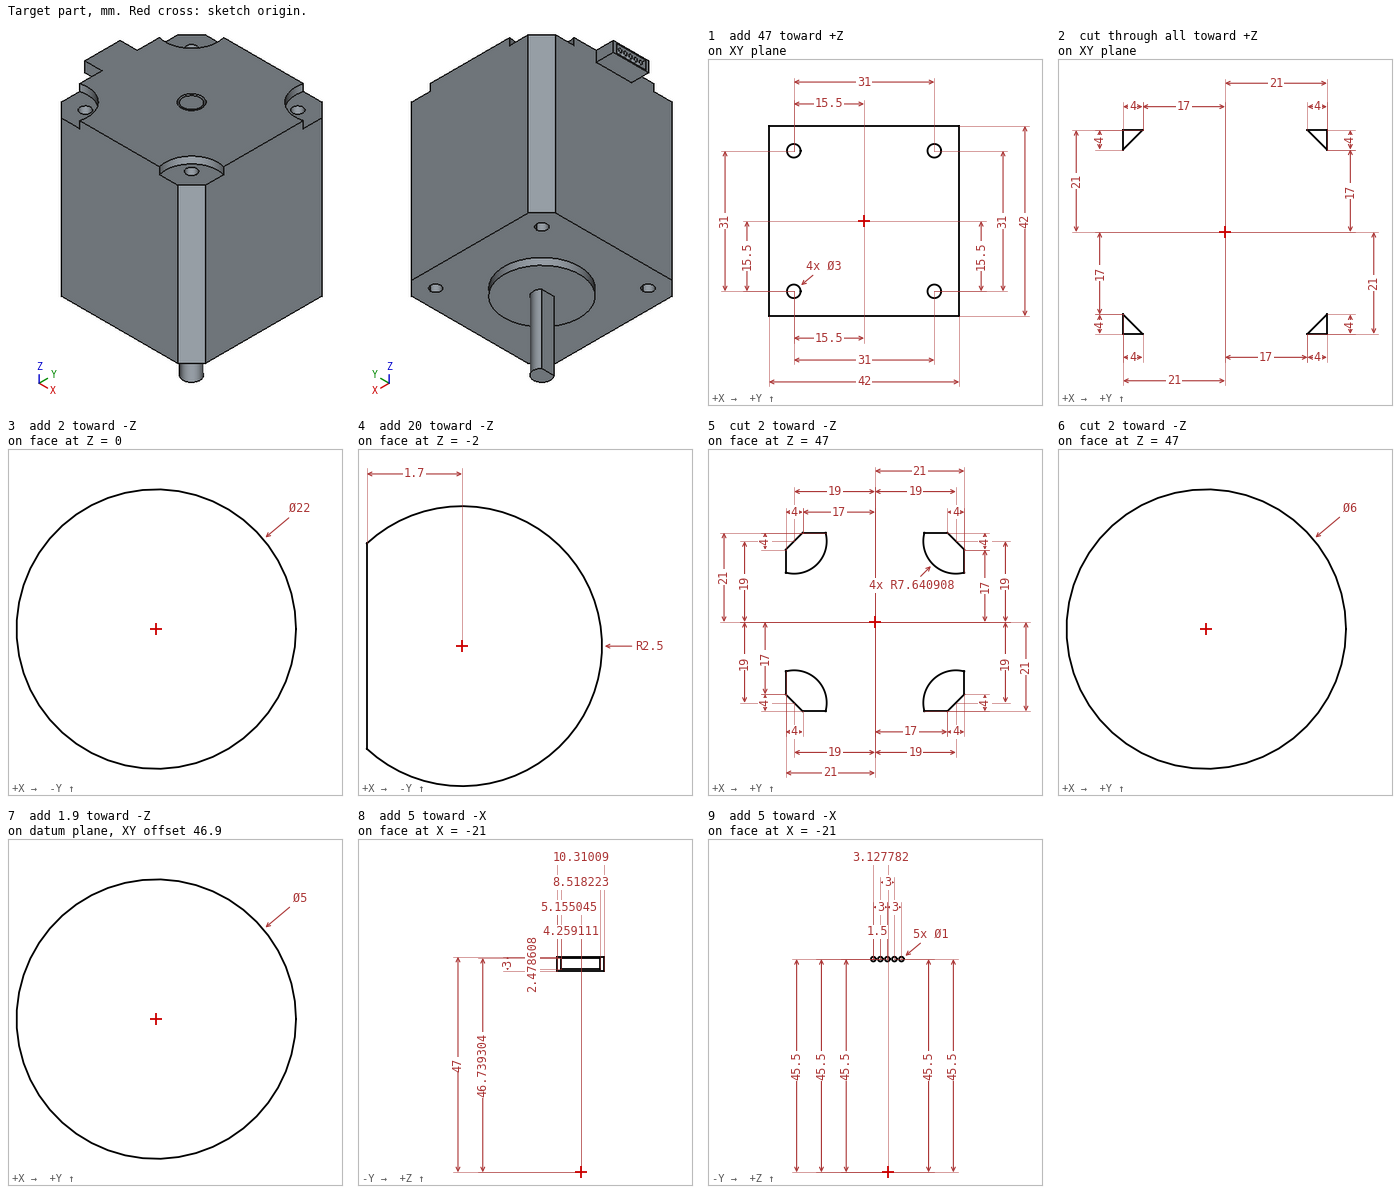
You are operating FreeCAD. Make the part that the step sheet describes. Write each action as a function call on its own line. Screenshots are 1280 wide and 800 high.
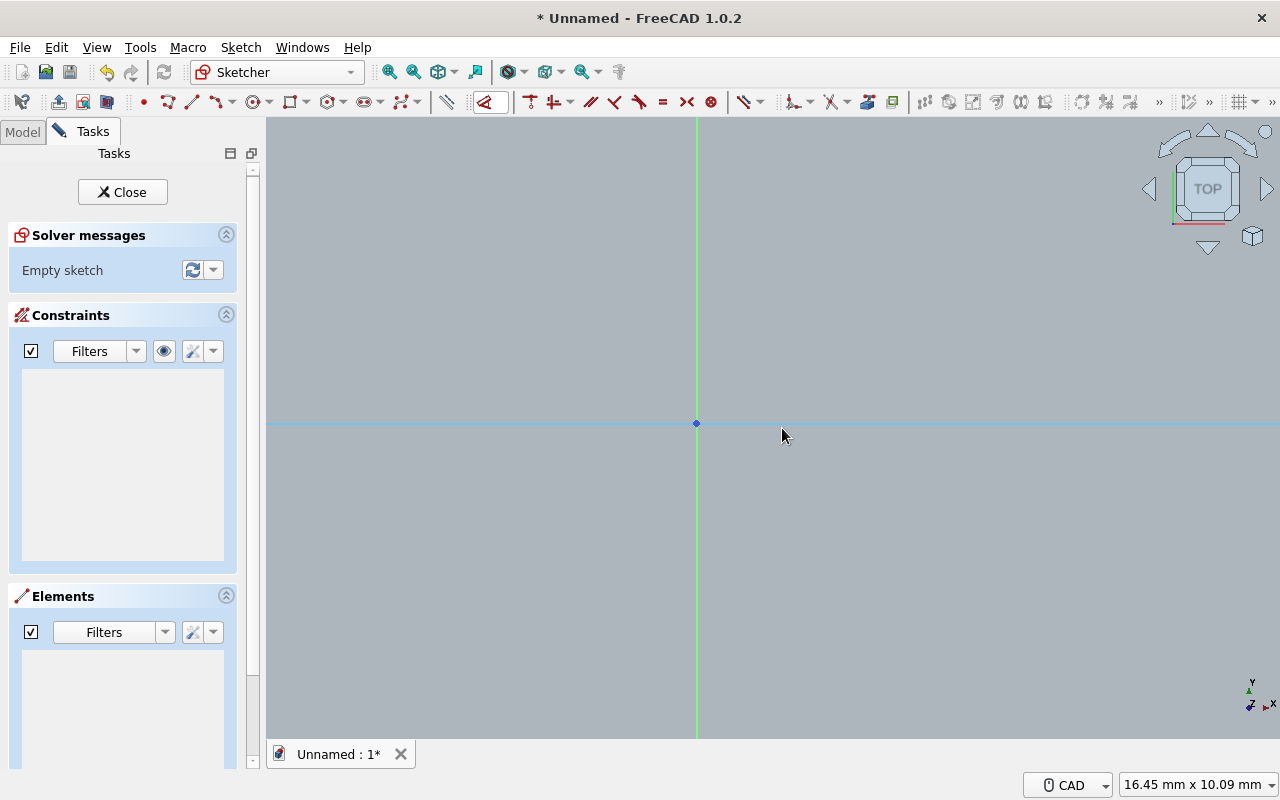
click(254, 102)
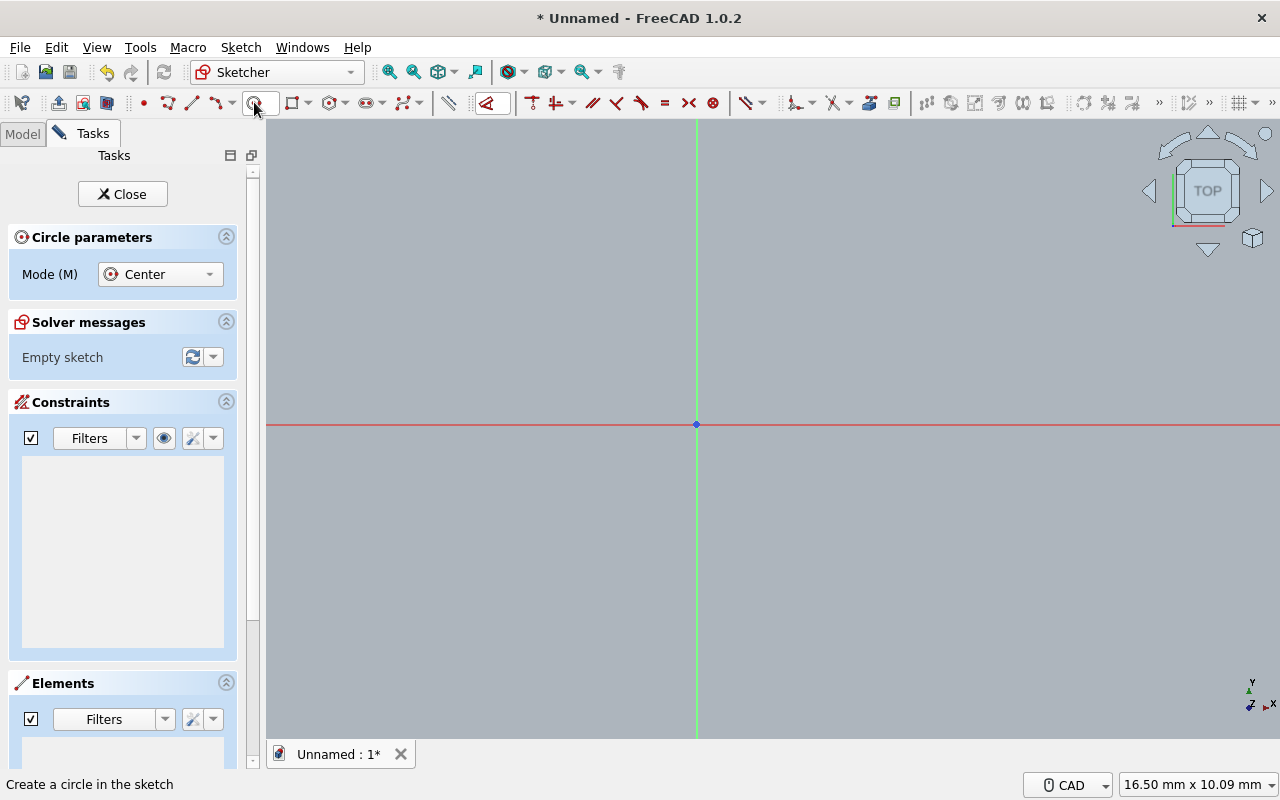
click(697, 425)
click(827, 295)
key(Escape)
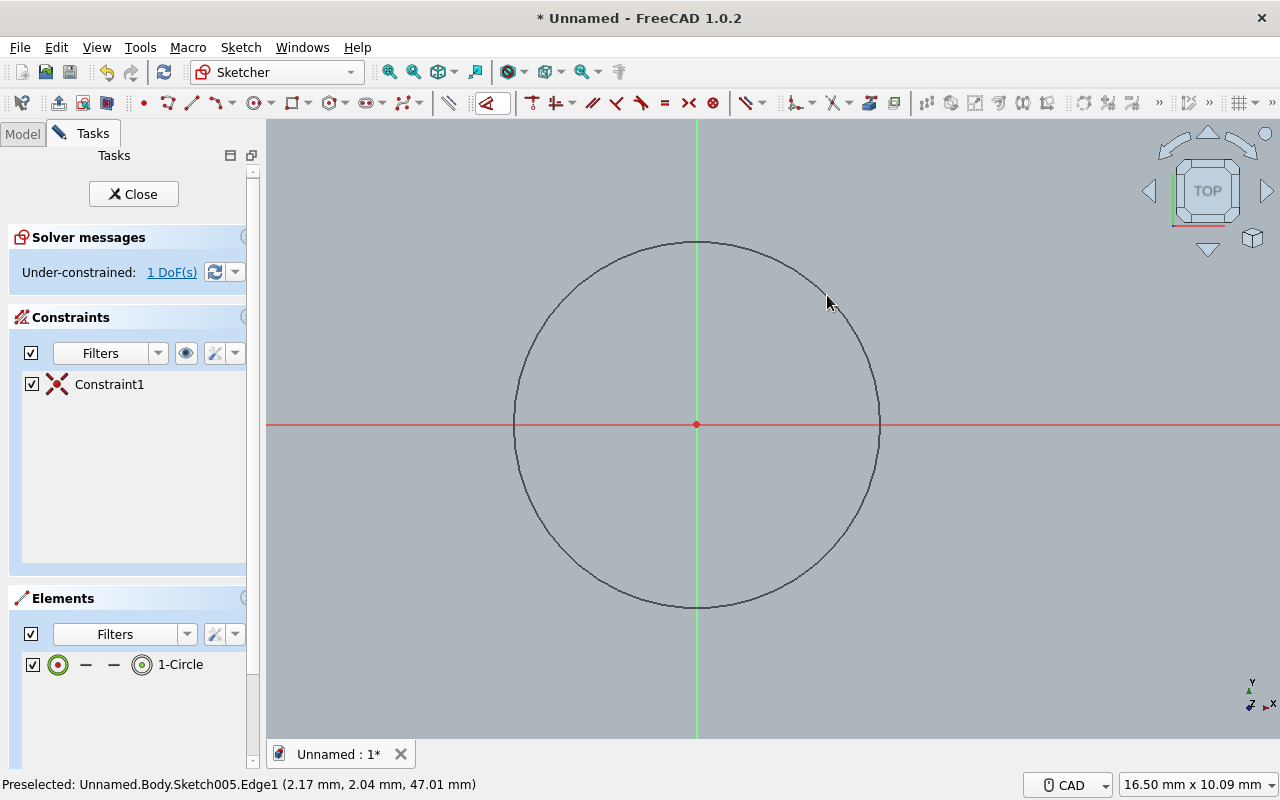
click(826, 295)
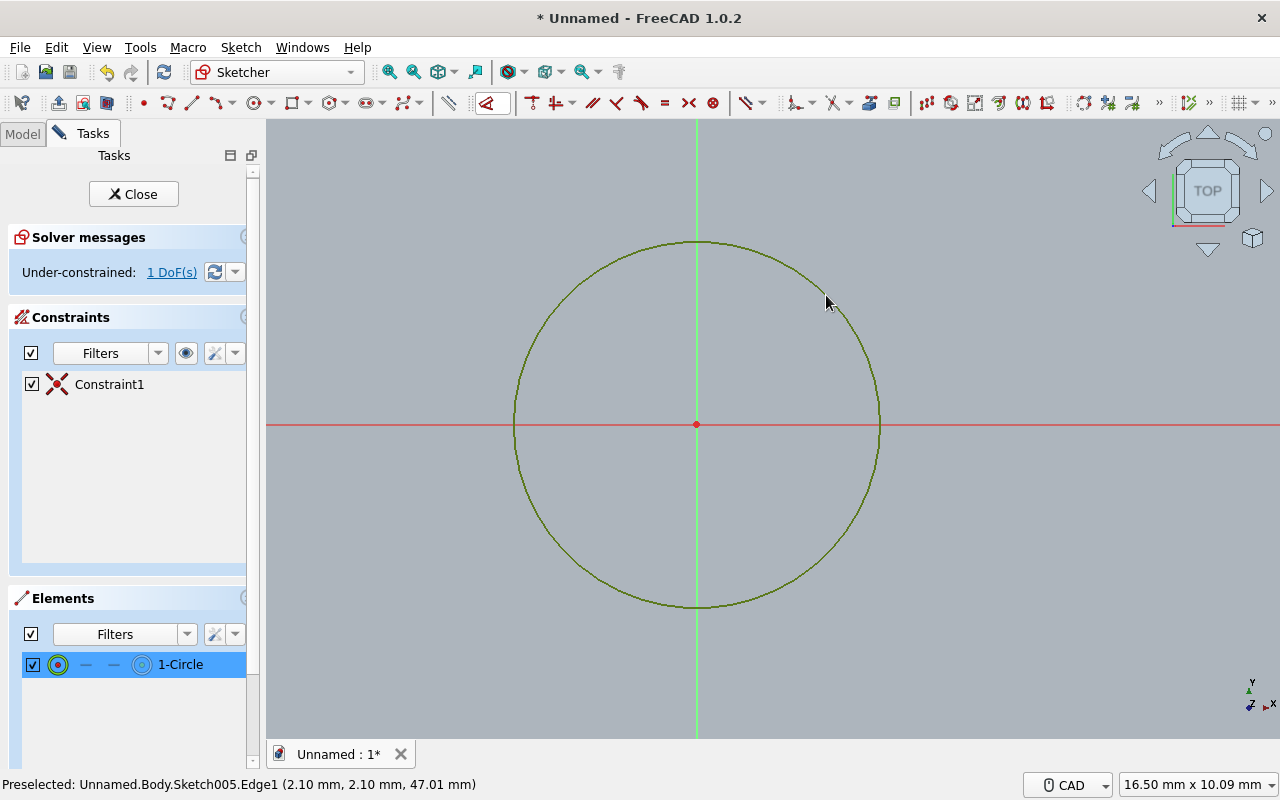
click(504, 104)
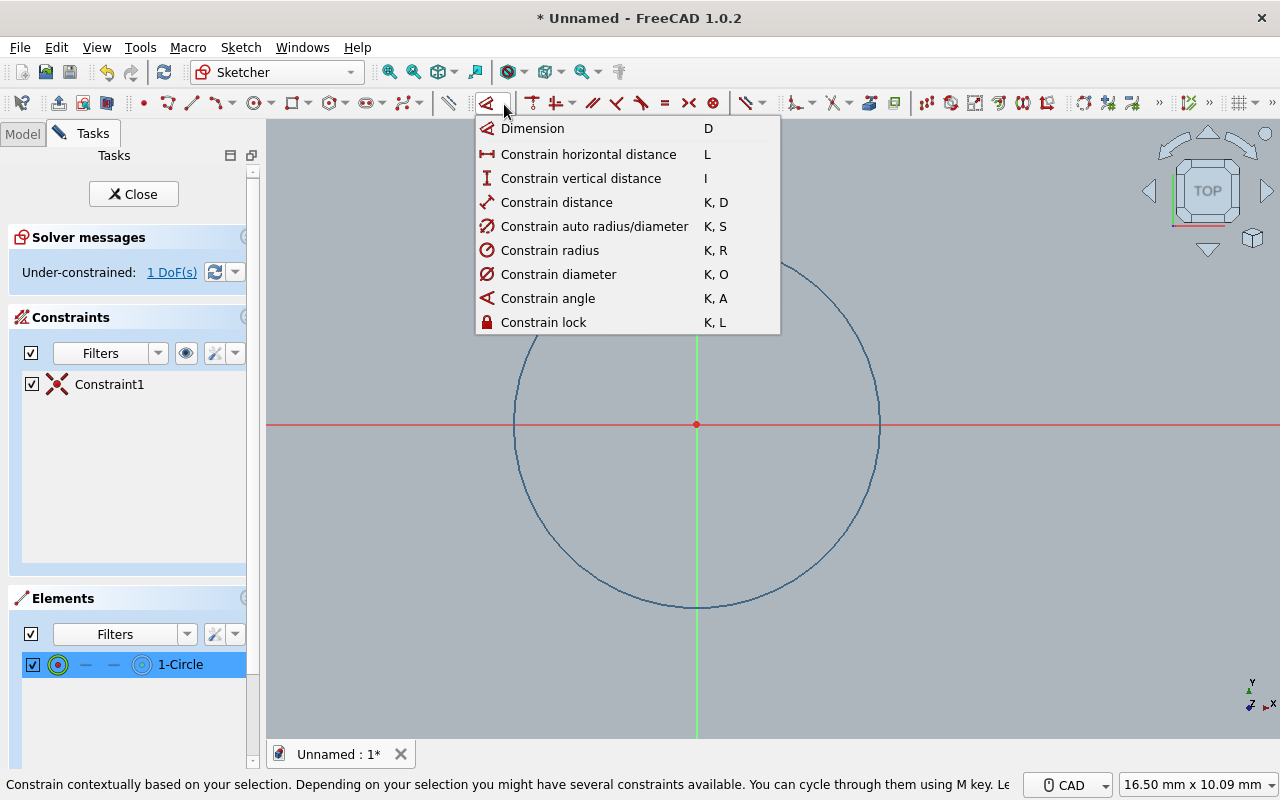
click(628, 274)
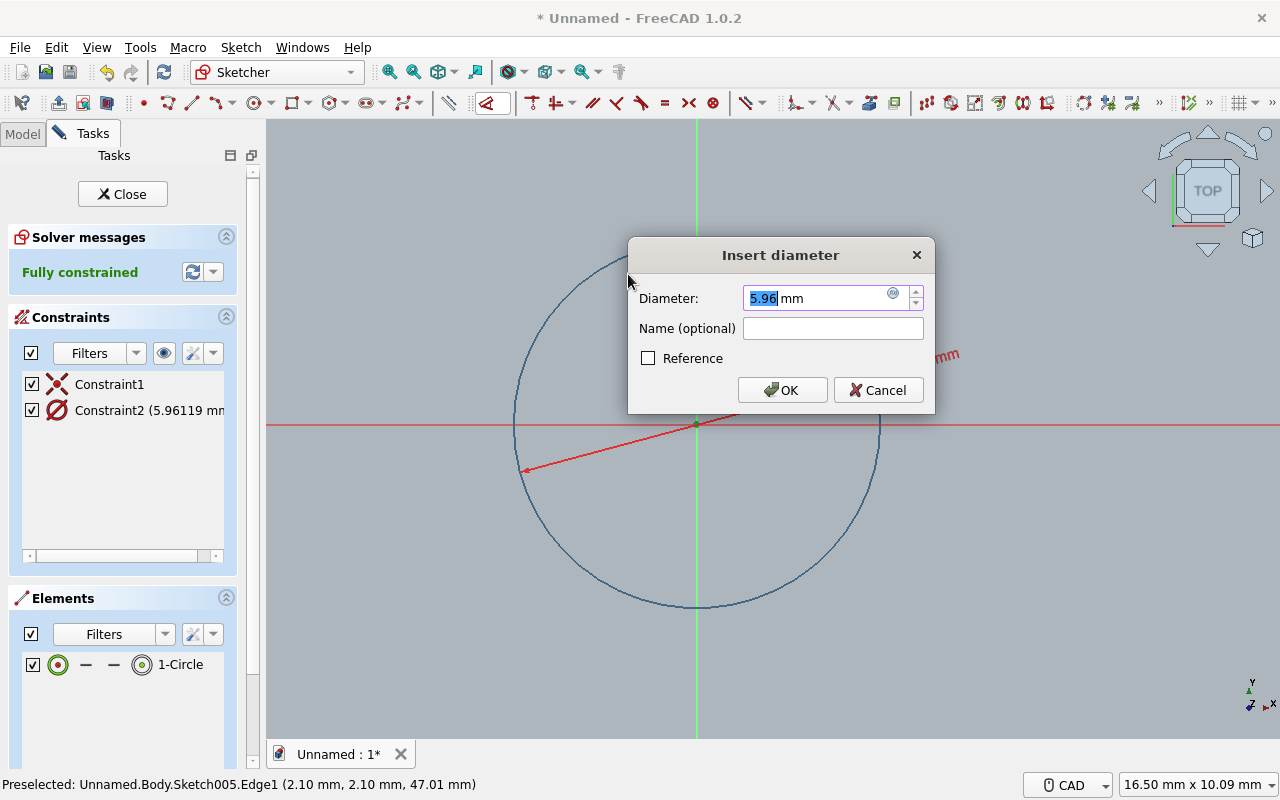
text(6)
key(Return)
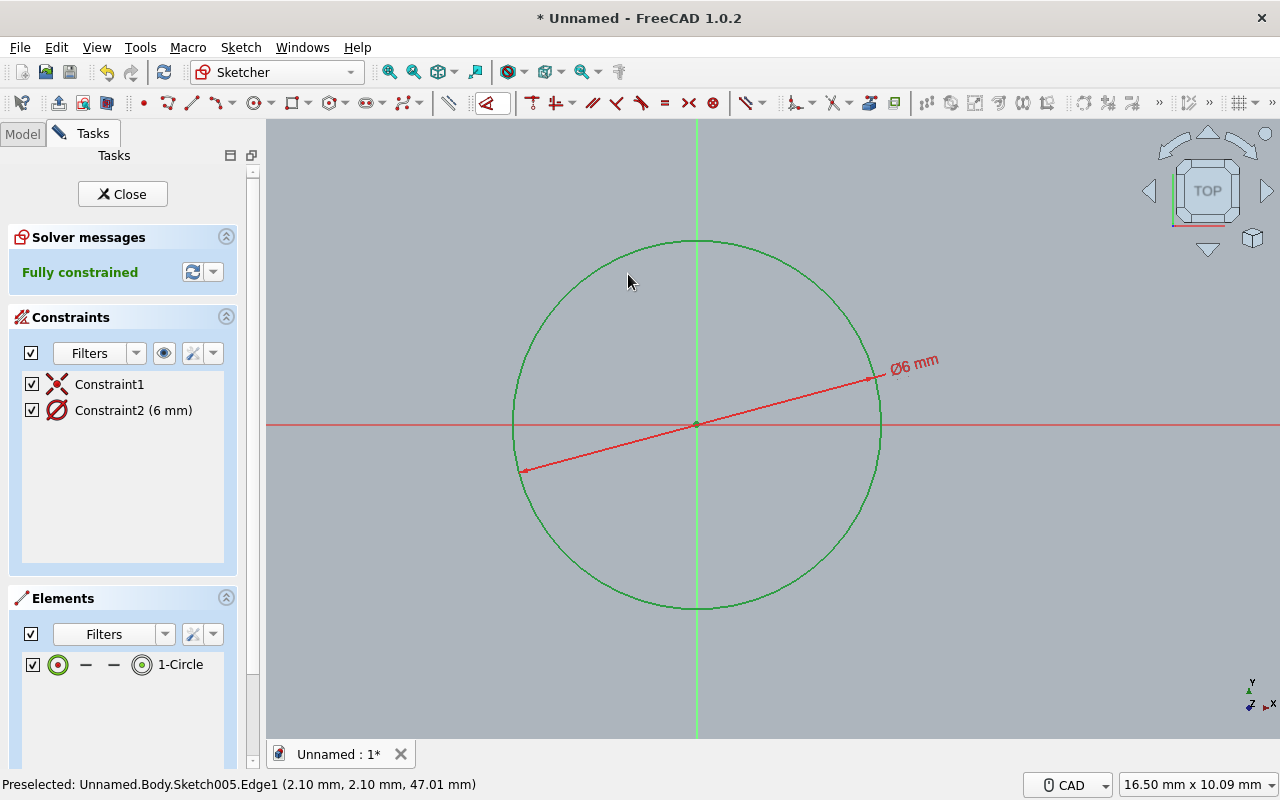
click(123, 194)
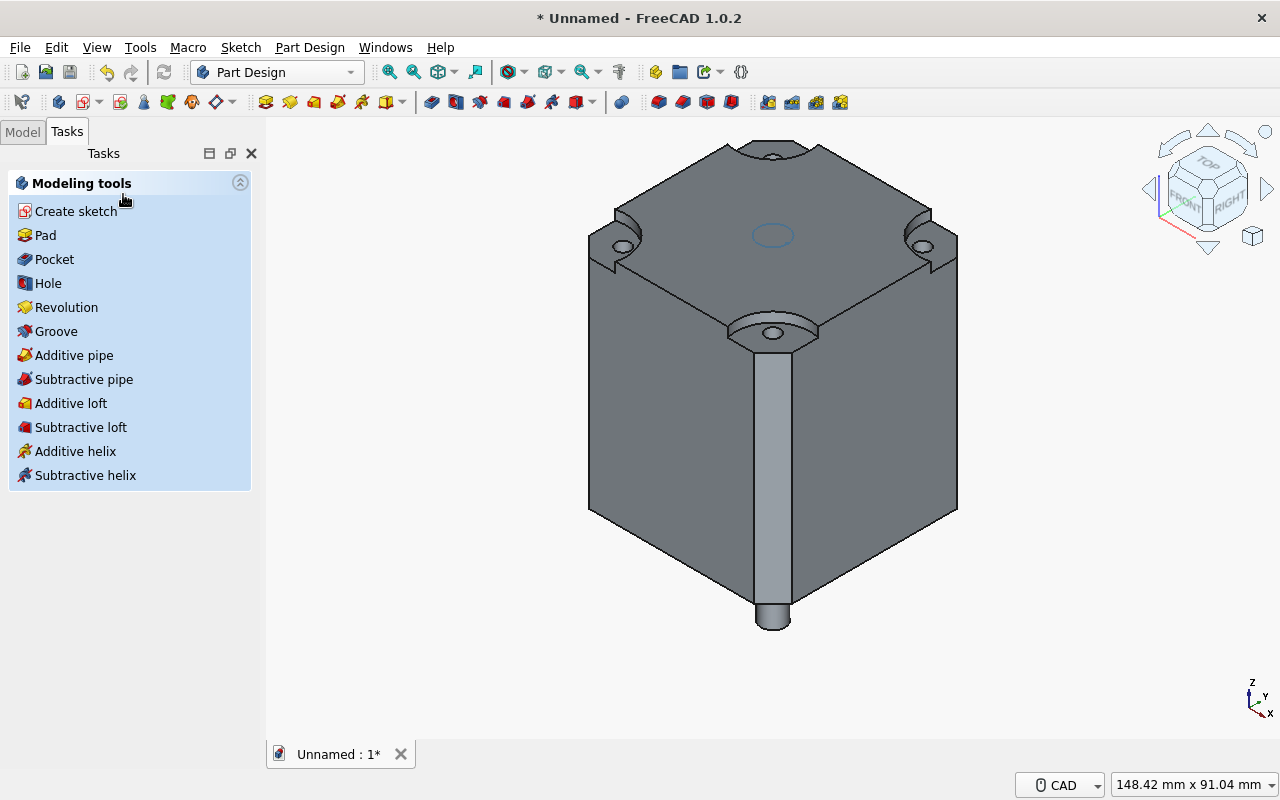
click(432, 102)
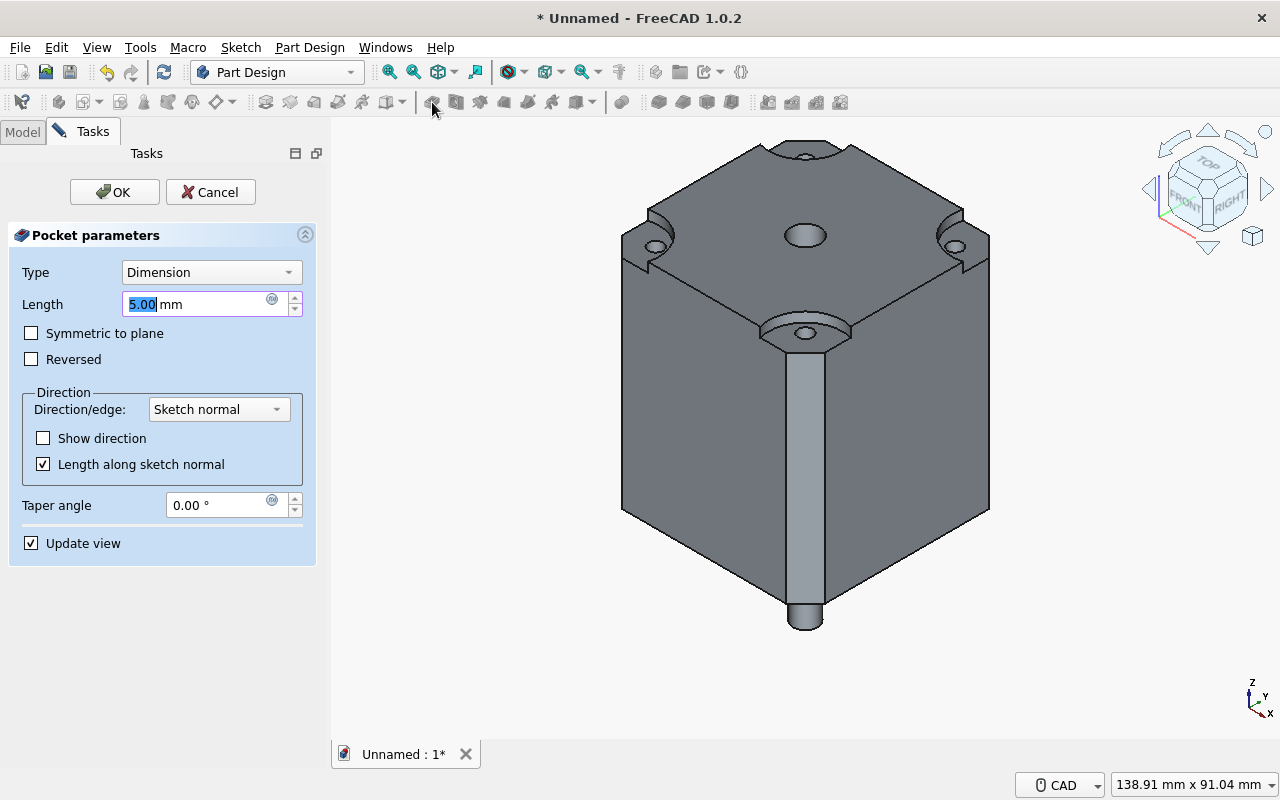
text(2)
key(Tab)